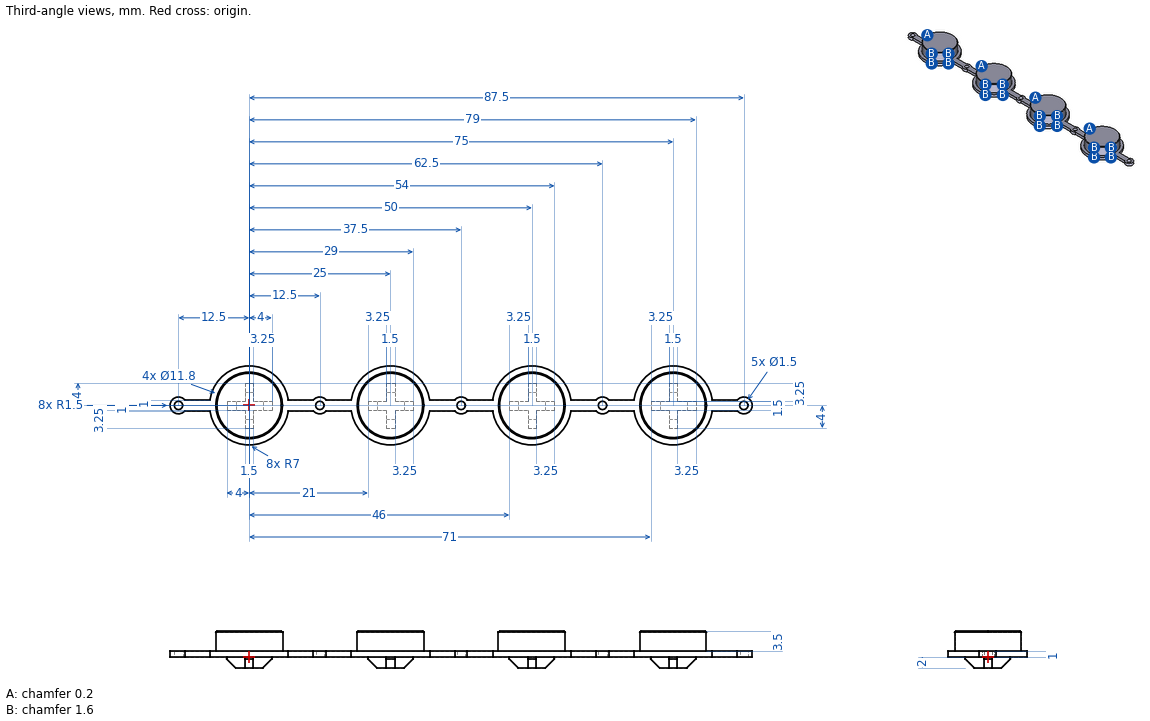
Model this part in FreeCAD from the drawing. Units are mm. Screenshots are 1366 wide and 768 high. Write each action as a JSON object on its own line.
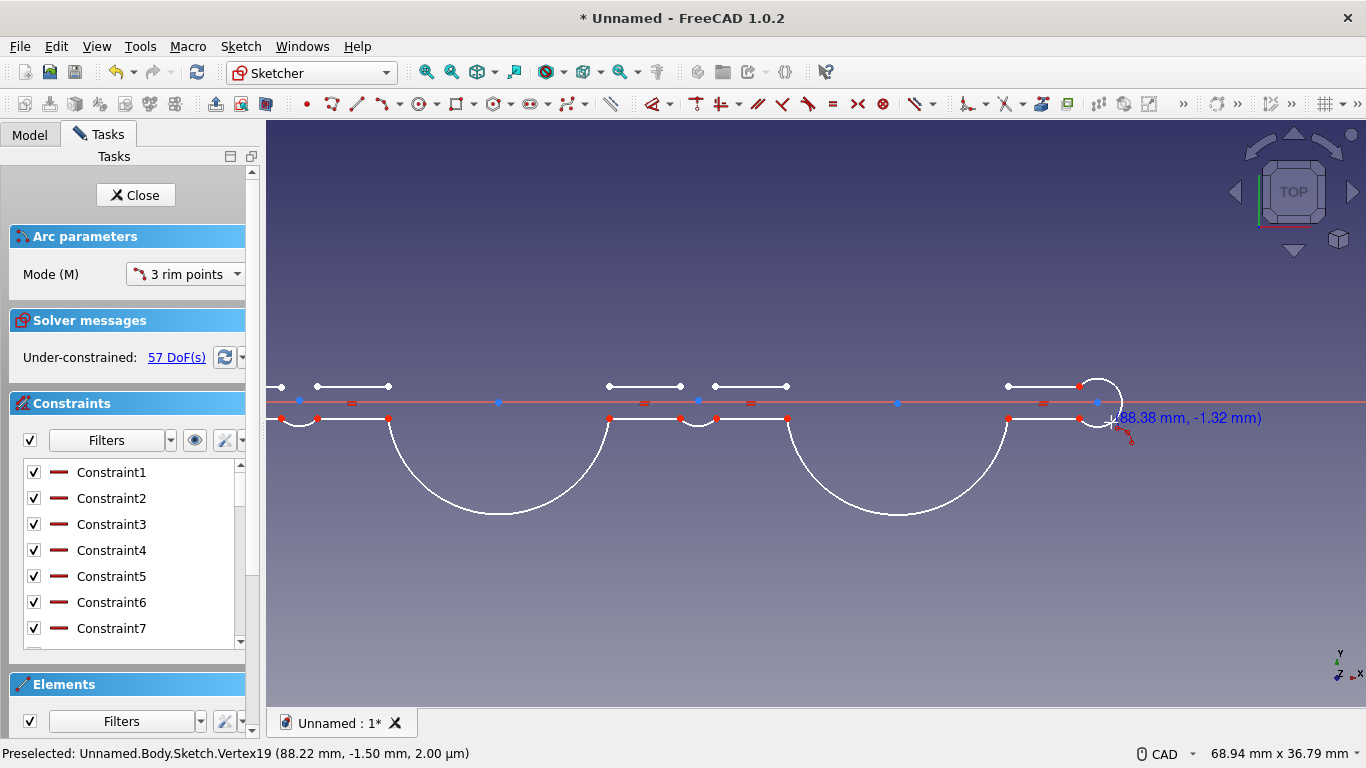
{"action": "left_click", "coordinate": [1009, 387]}
{"action": "left_click", "coordinate": [787, 387]}
{"action": "left_click", "coordinate": [898, 290]}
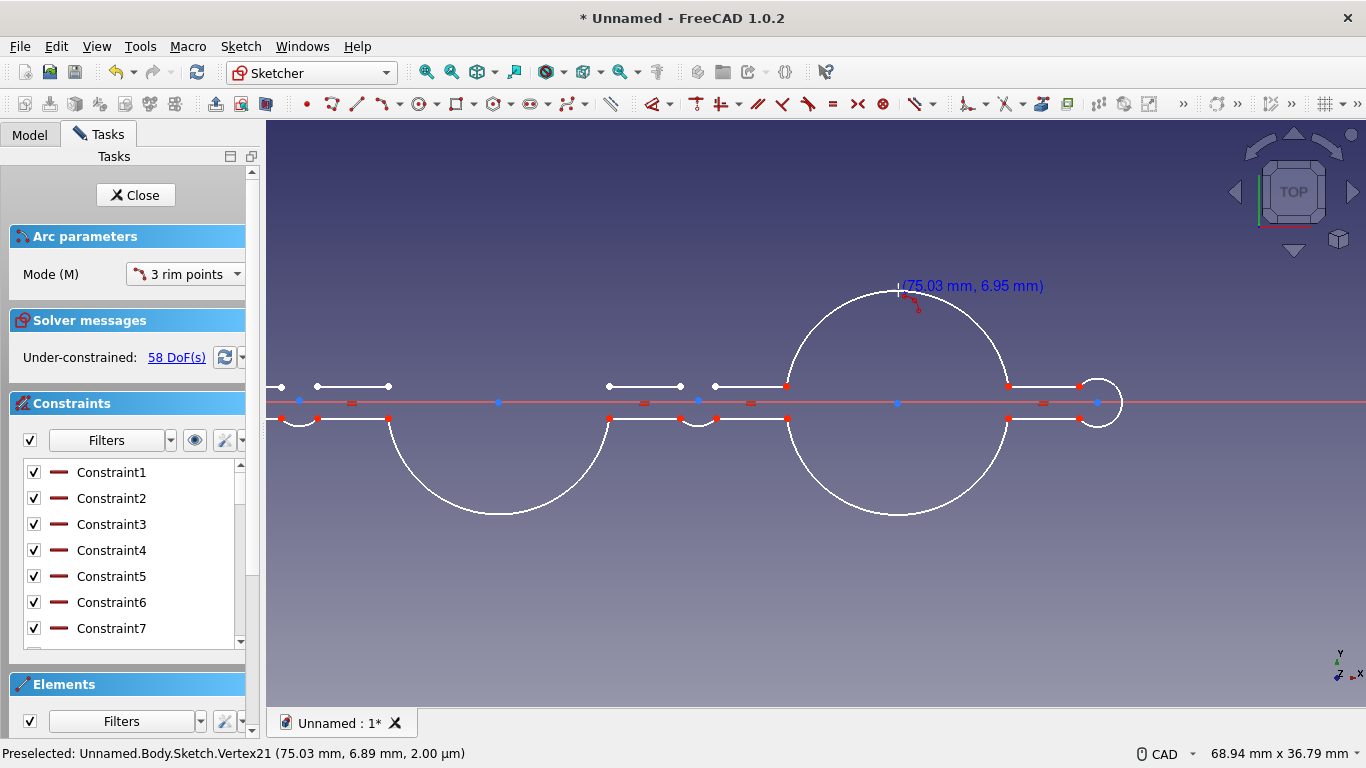
{"action": "left_click", "coordinate": [716, 387]}
{"action": "left_click", "coordinate": [681, 387]}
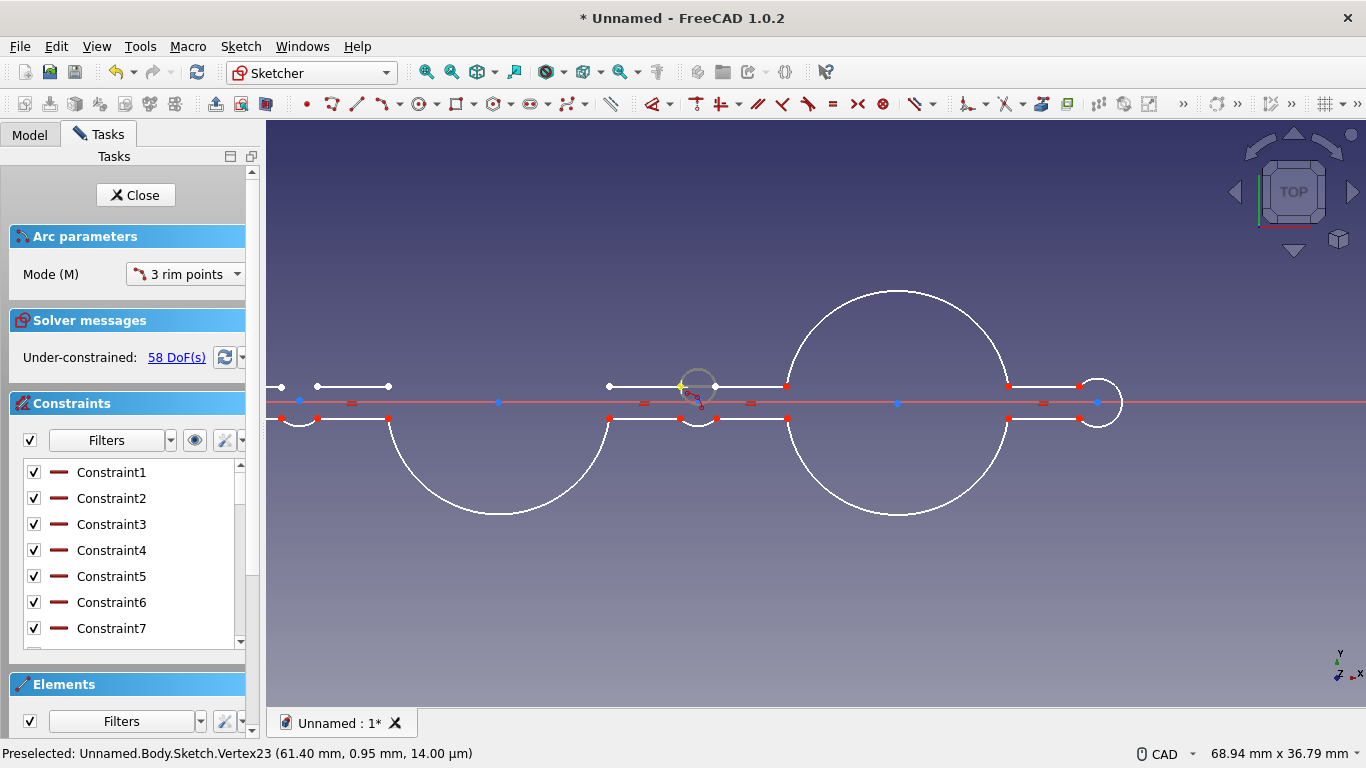
{"action": "scroll", "coordinate": [698, 378], "scroll_direction": "up", "scroll_amount": 4}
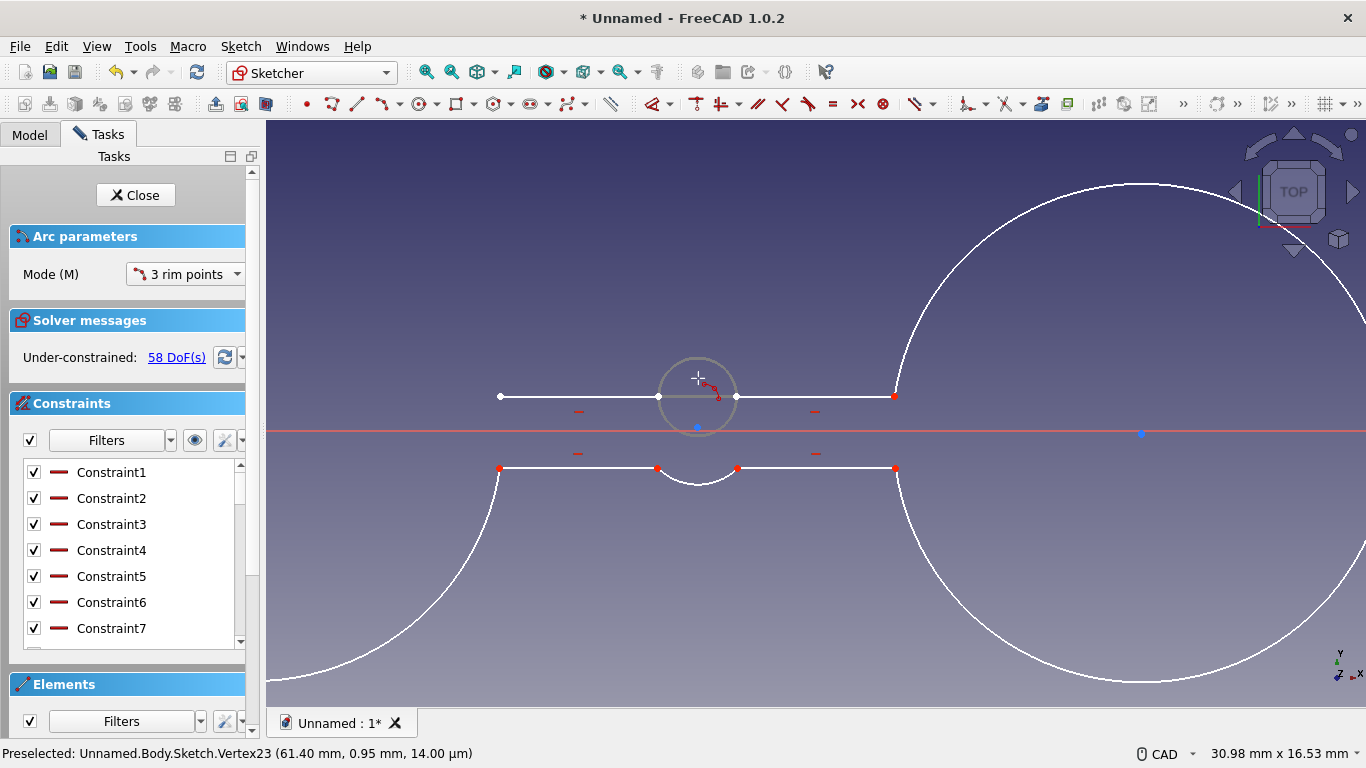
{"action": "left_click", "coordinate": [698, 377]}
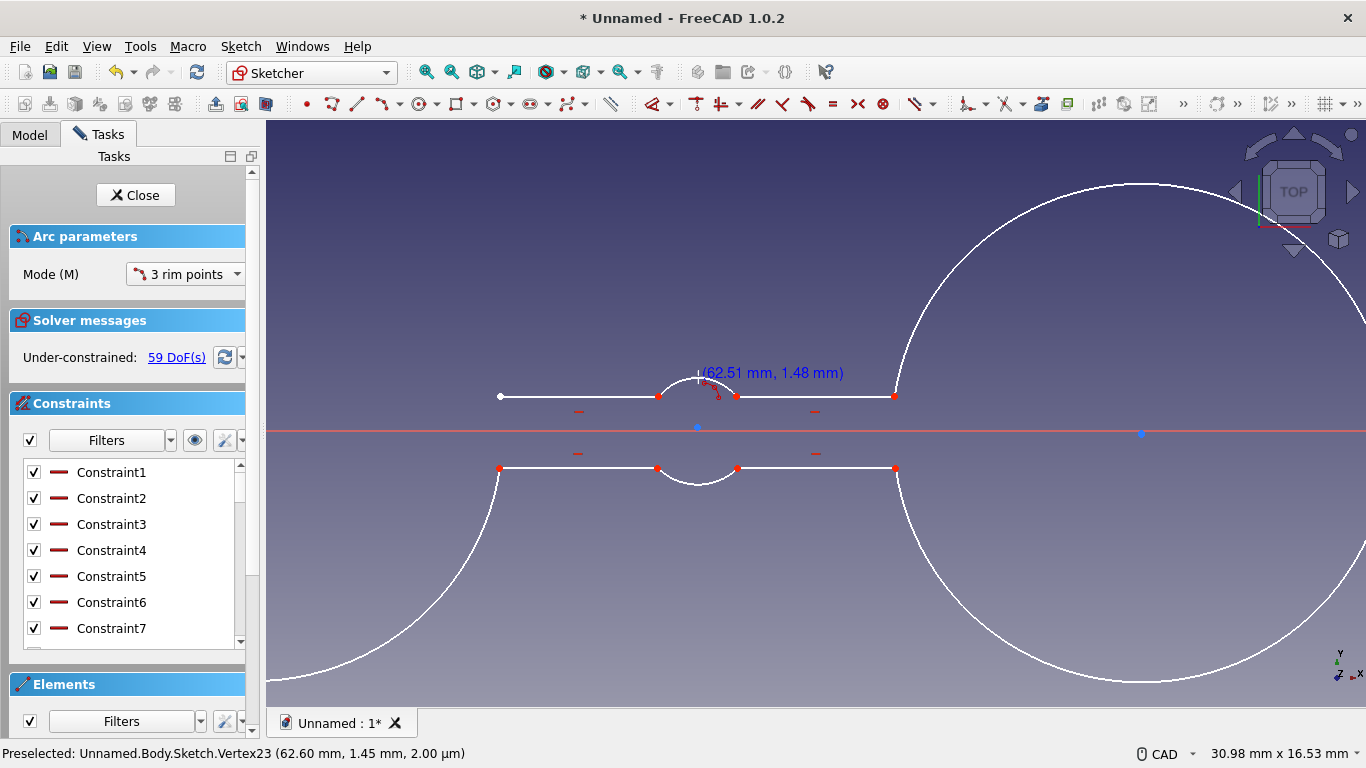
{"action": "left_click", "coordinate": [501, 397]}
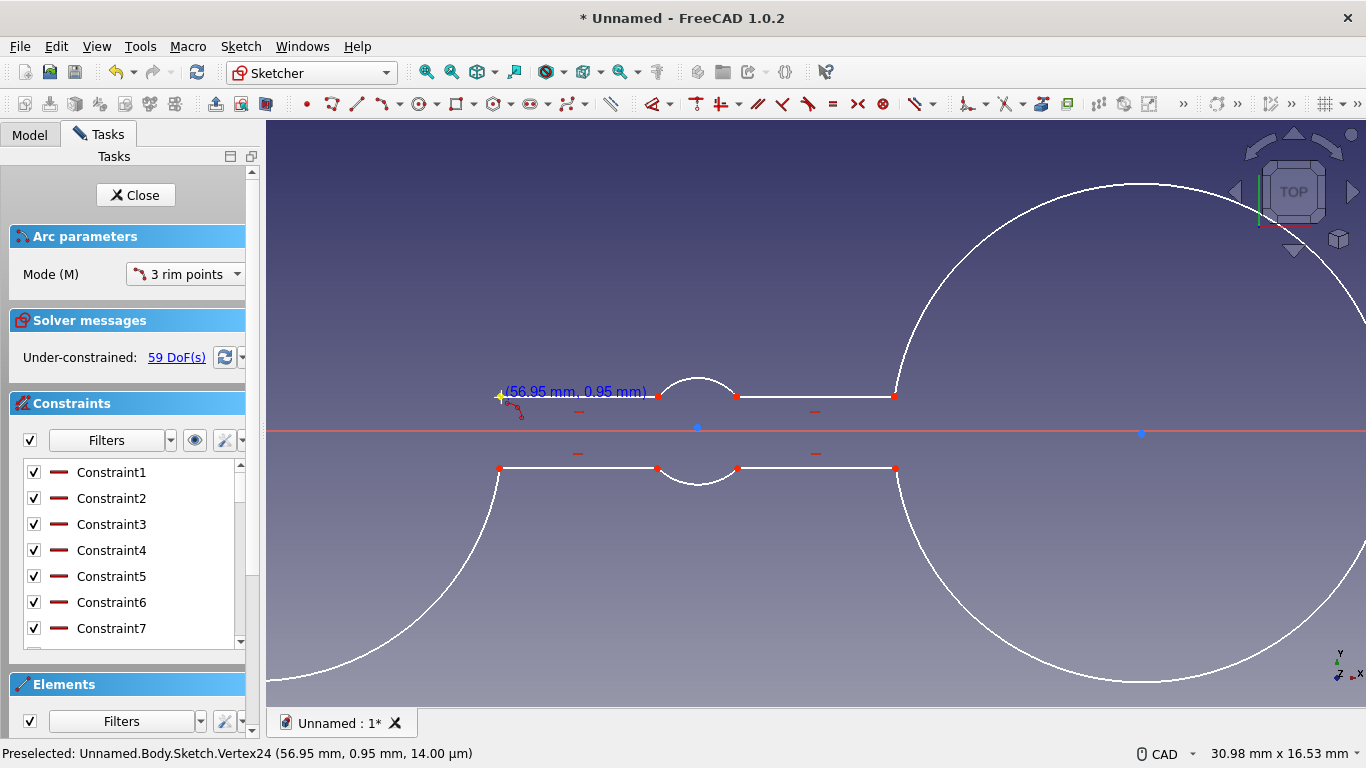
{"action": "scroll", "coordinate": [933, 410], "scroll_direction": "down", "scroll_amount": 9}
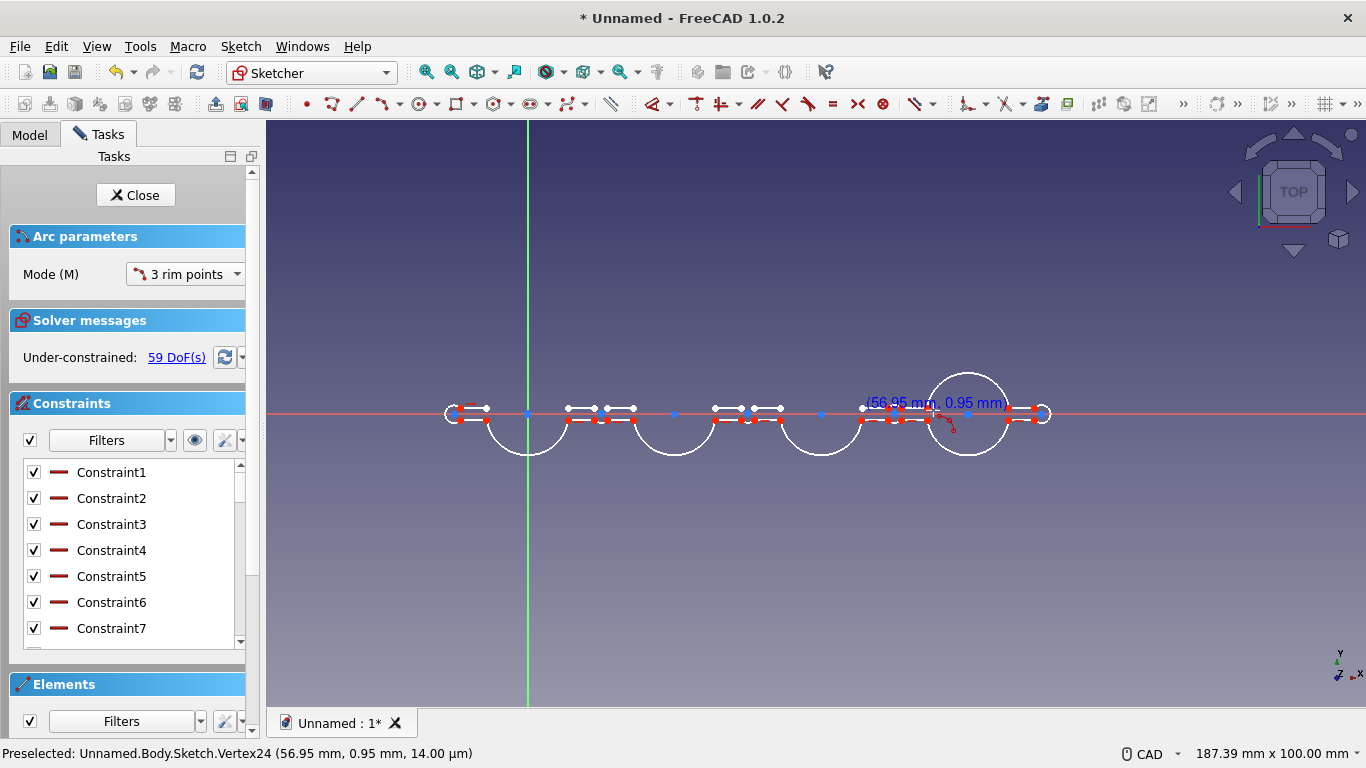
{"action": "scroll", "coordinate": [781, 408], "scroll_direction": "up", "scroll_amount": 5}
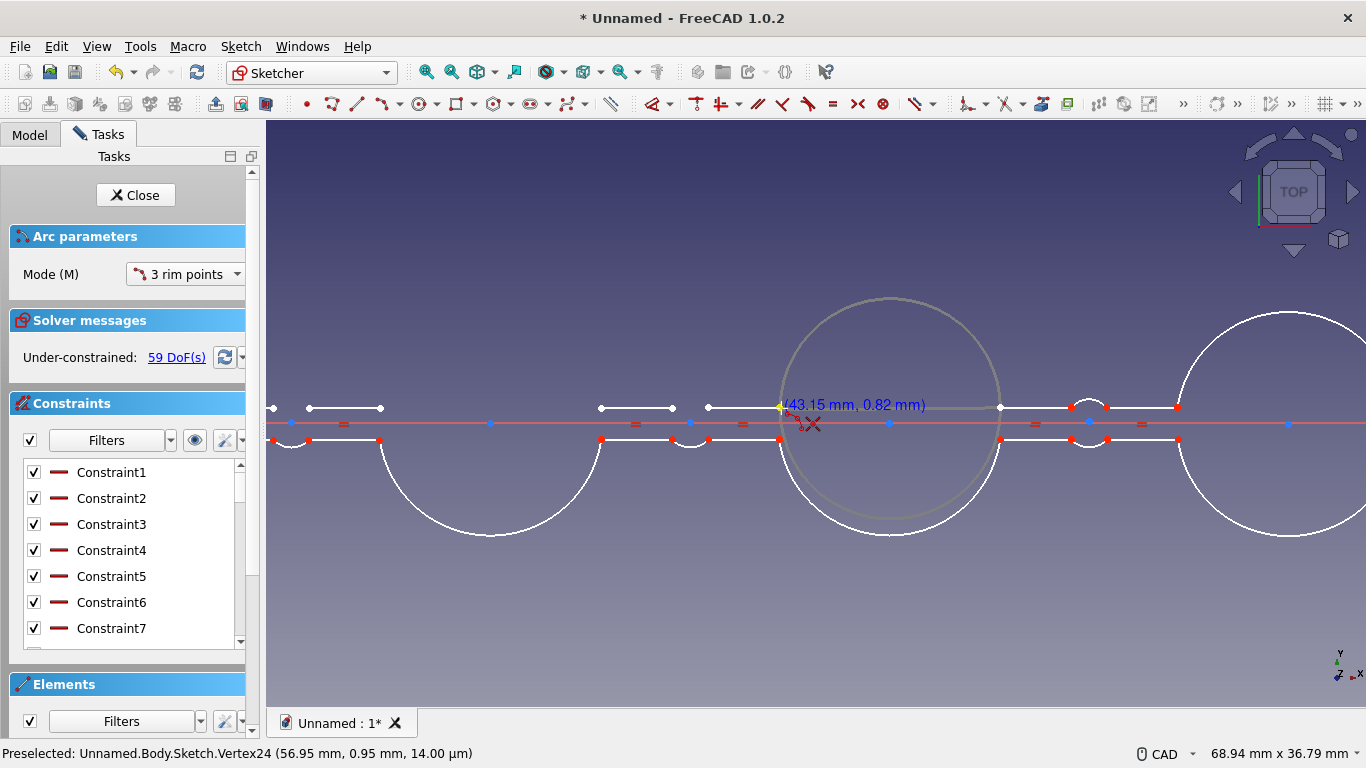
{"action": "left_click", "coordinate": [780, 408]}
{"action": "left_click", "coordinate": [890, 311]}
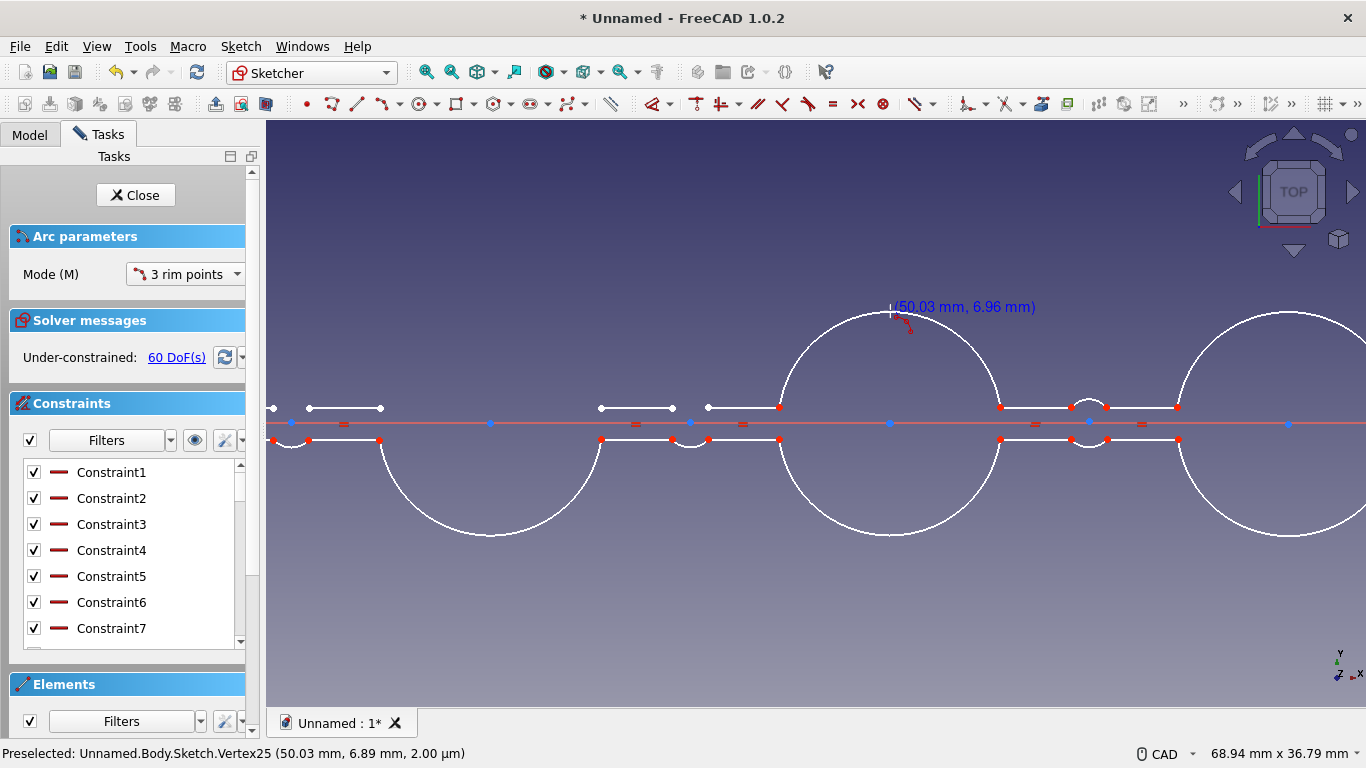
{"action": "left_click", "coordinate": [708, 408]}
{"action": "left_click", "coordinate": [672, 408]}